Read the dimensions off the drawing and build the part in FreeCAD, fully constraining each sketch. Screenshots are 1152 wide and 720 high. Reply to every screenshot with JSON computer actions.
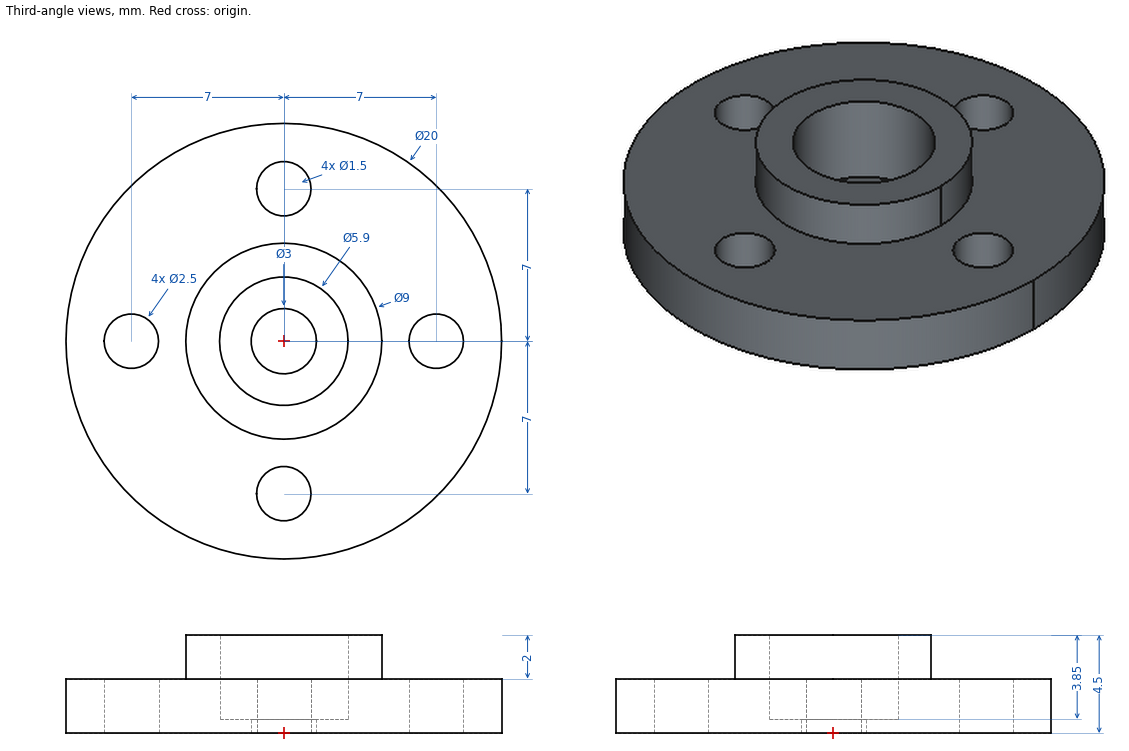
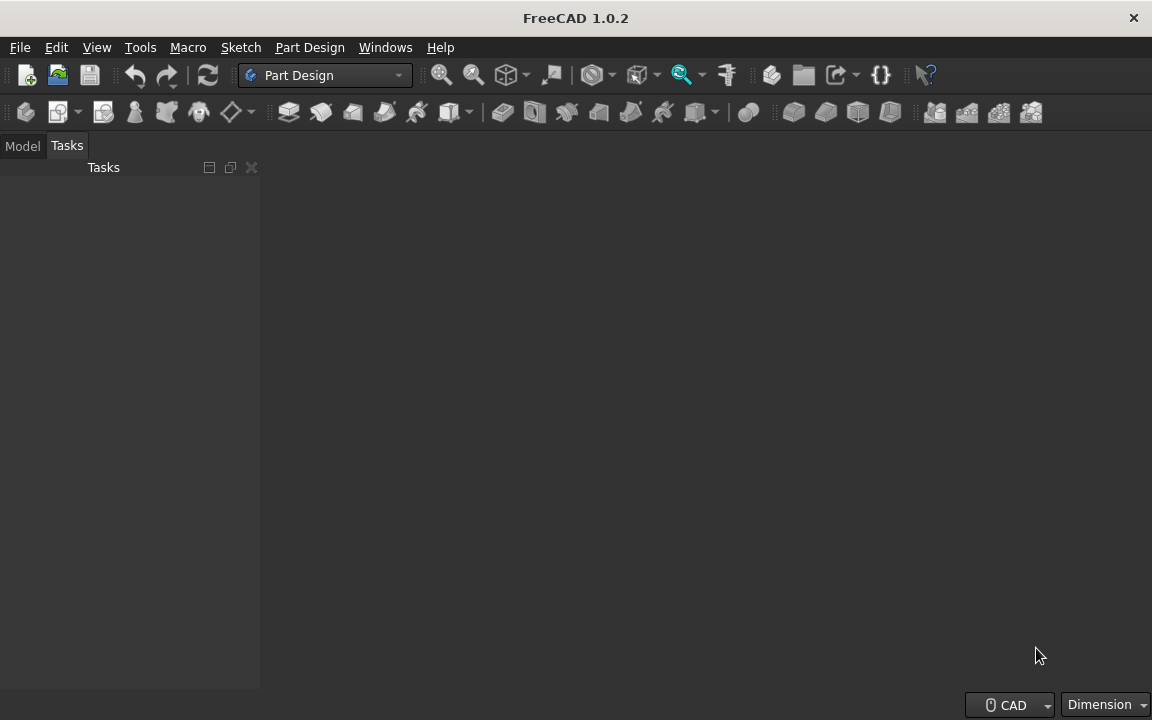
{"action": "left_click", "coordinate": [26, 76]}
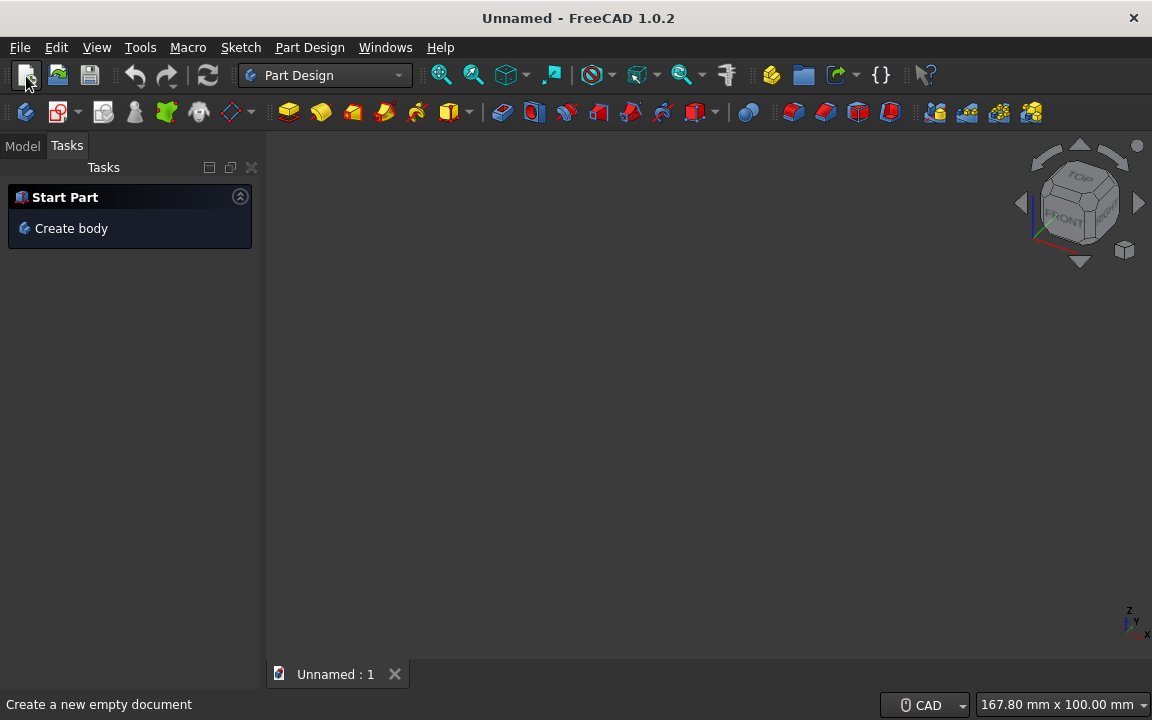
{"action": "left_click", "coordinate": [58, 112]}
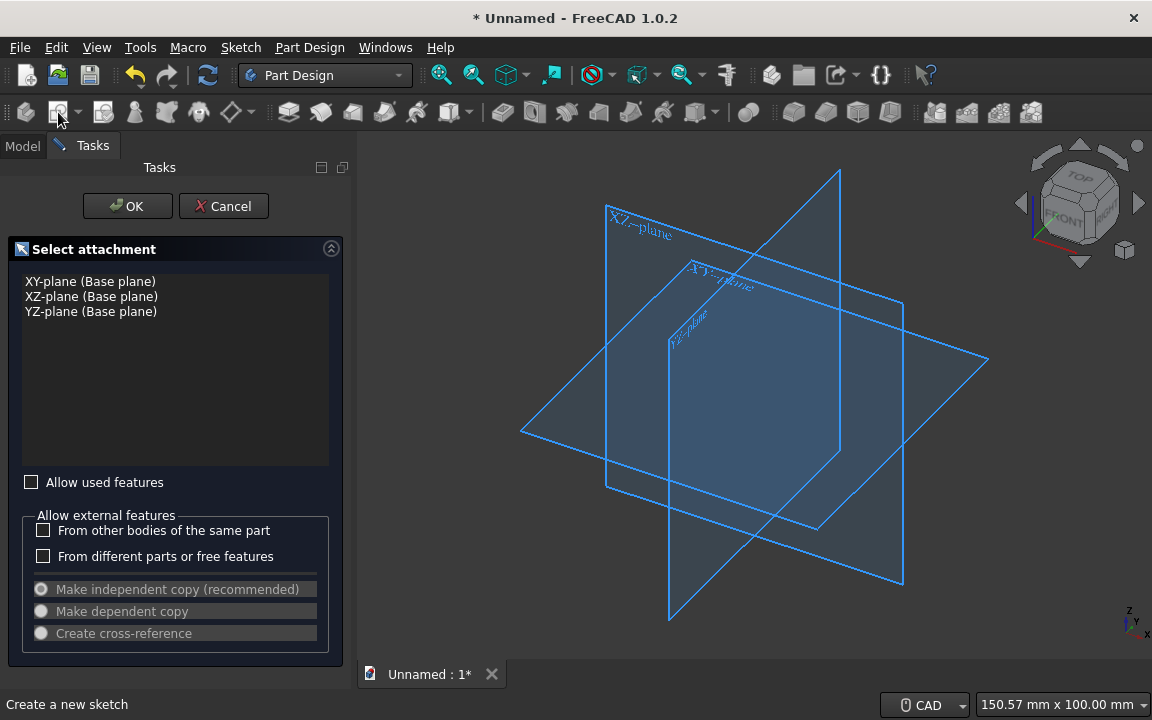
{"action": "left_click", "coordinate": [82, 282]}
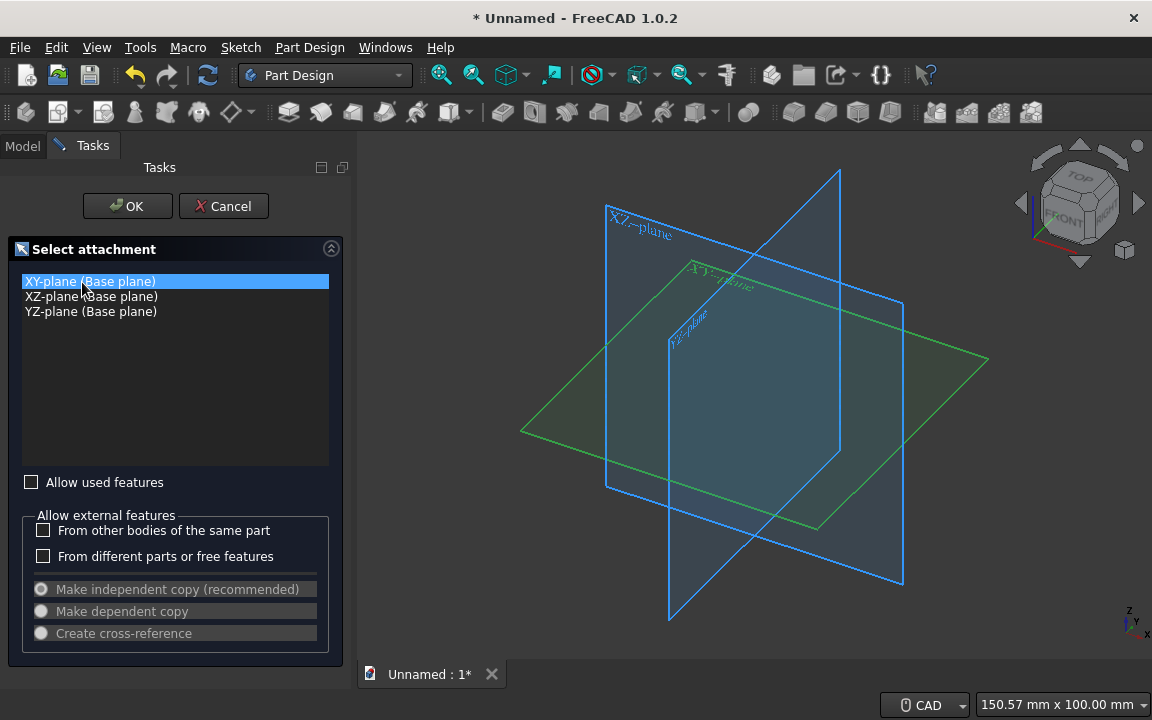
{"action": "left_click", "coordinate": [128, 206]}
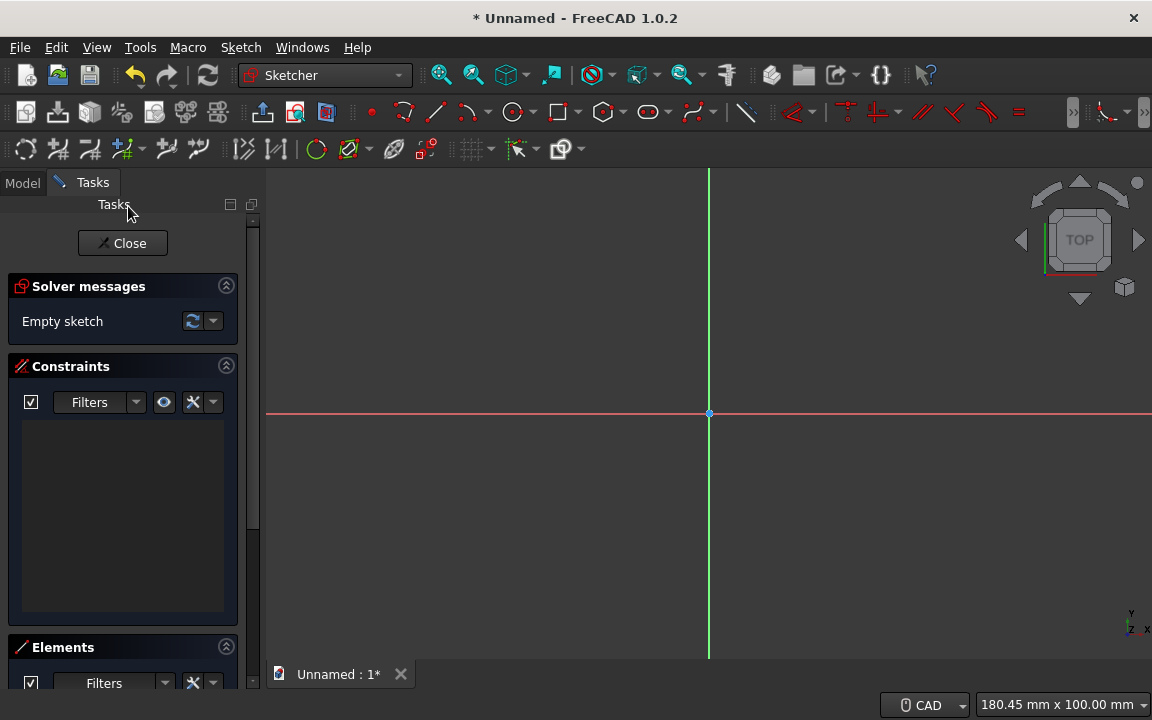
{"action": "scroll", "coordinate": [739, 414], "scroll_direction": "up", "scroll_amount": 6}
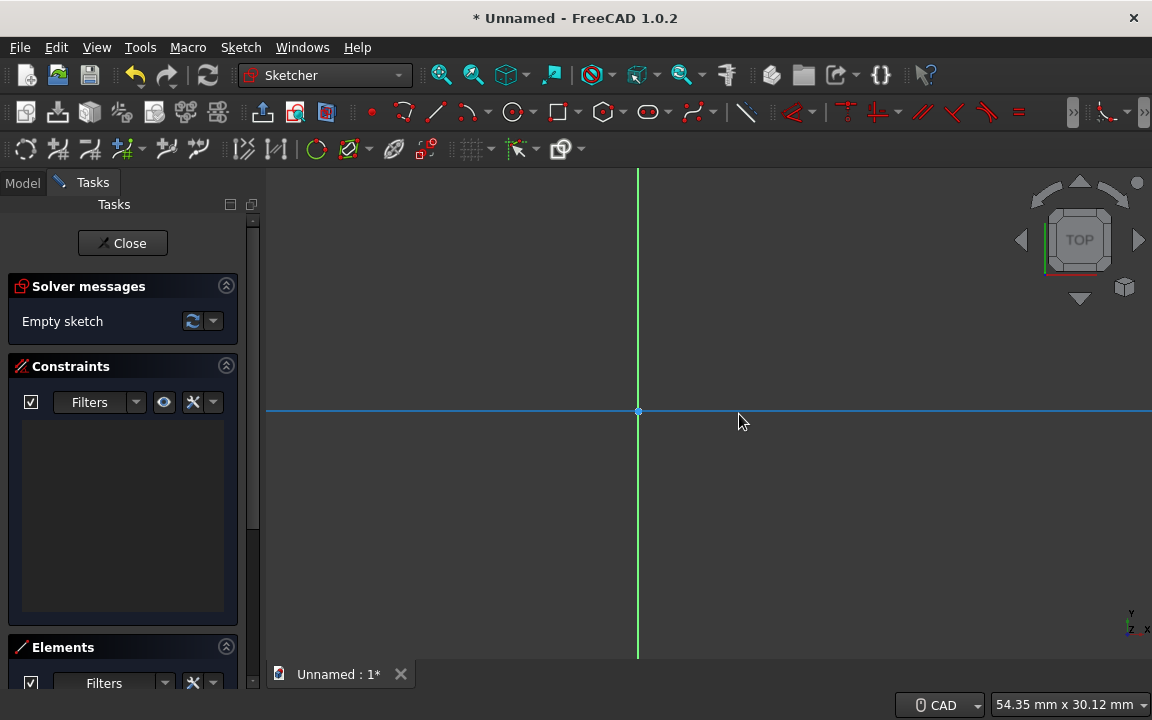
{"action": "key", "text": "g c"}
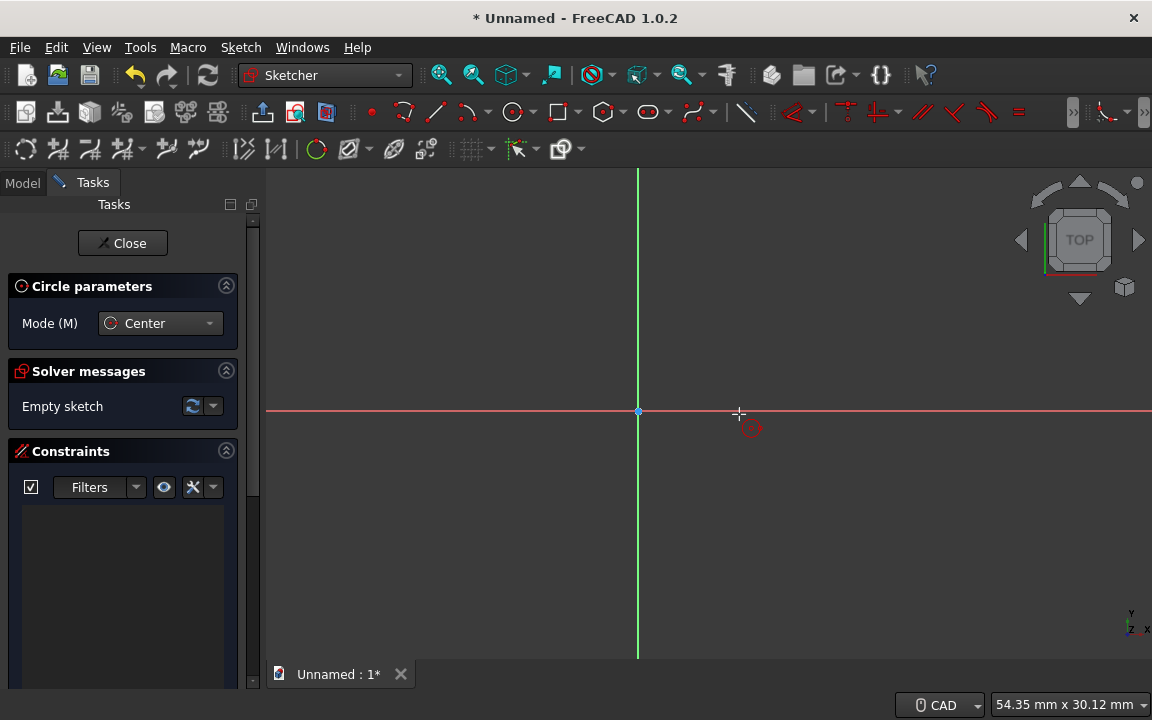
{"action": "left_click", "coordinate": [638, 411]}
{"action": "left_click", "coordinate": [753, 296]}
{"action": "key", "text": "Escape"}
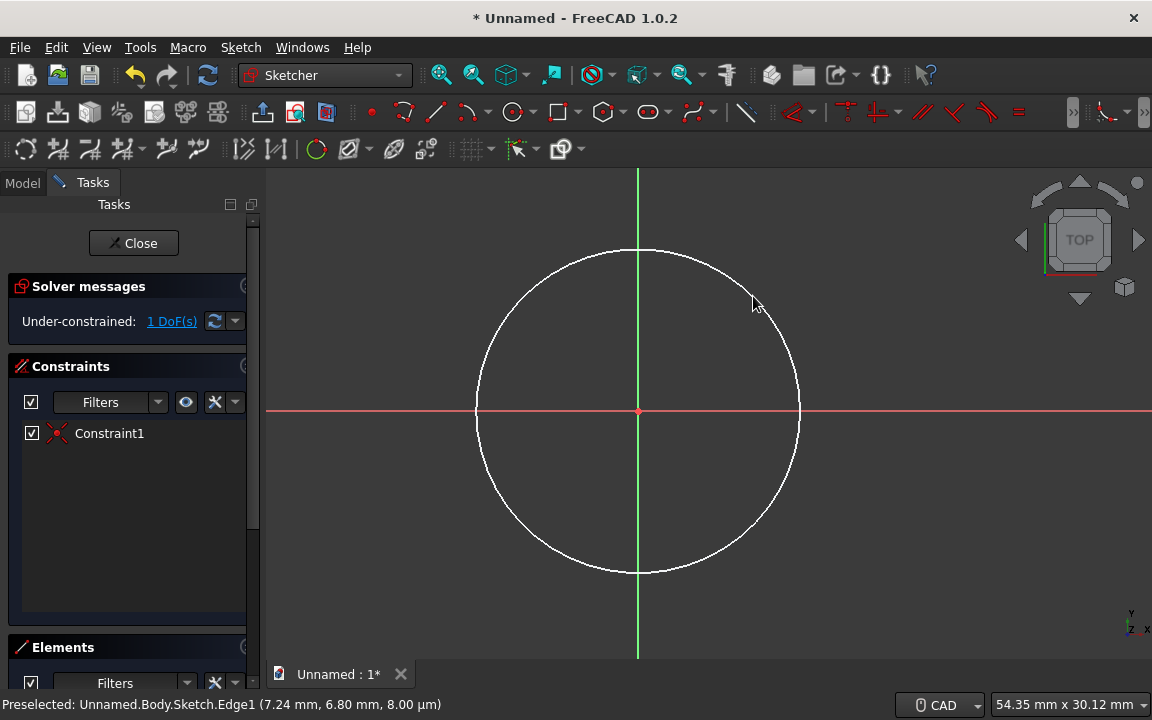
{"action": "key", "text": "d"}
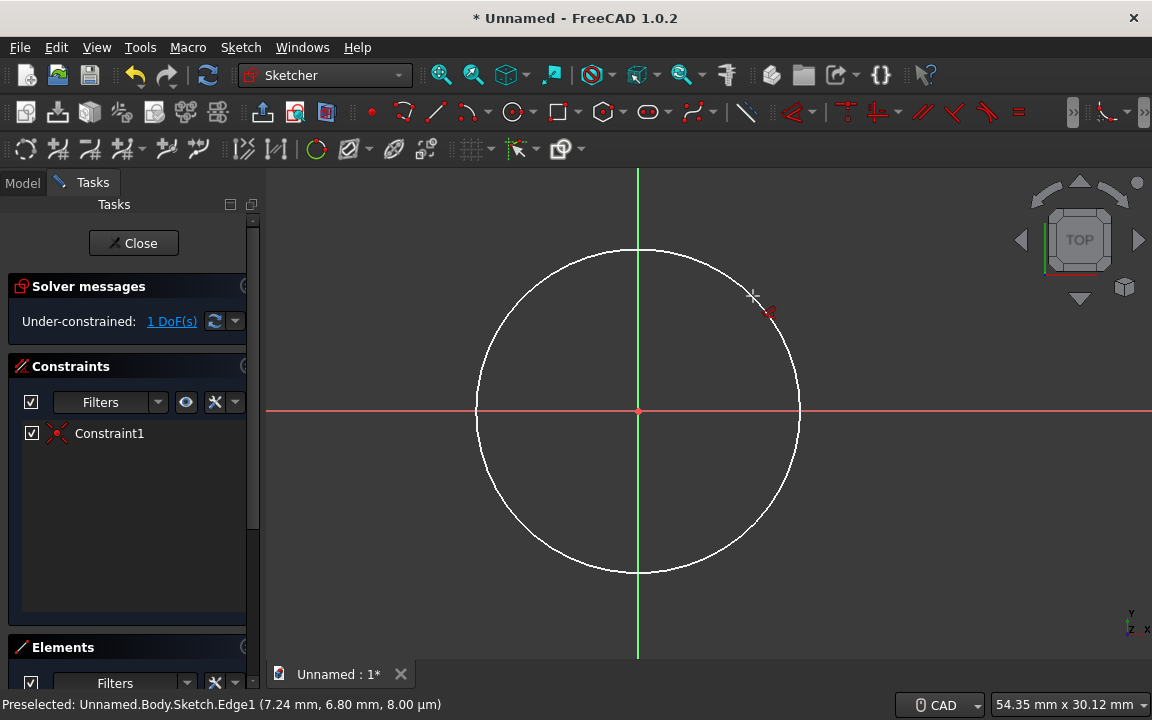
{"action": "left_click", "coordinate": [752, 296]}
{"action": "left_click", "coordinate": [774, 273]}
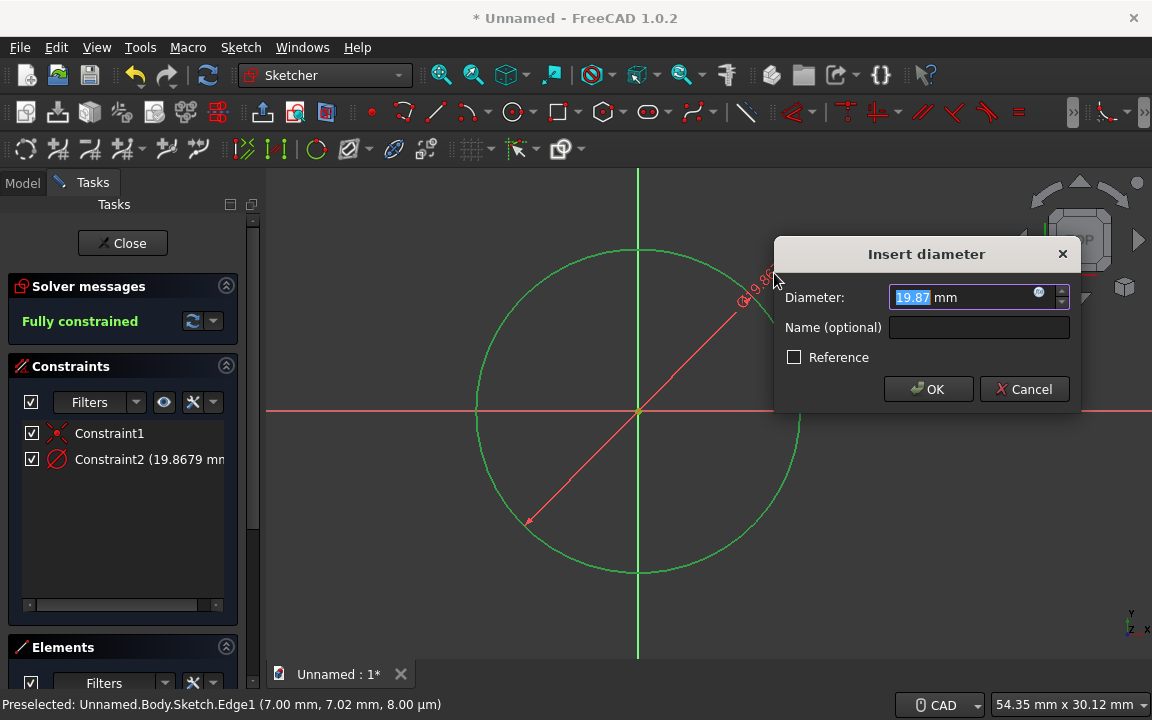
{"action": "type", "text": "20"}
{"action": "key", "text": "Return"}
{"action": "key", "text": "Escape"}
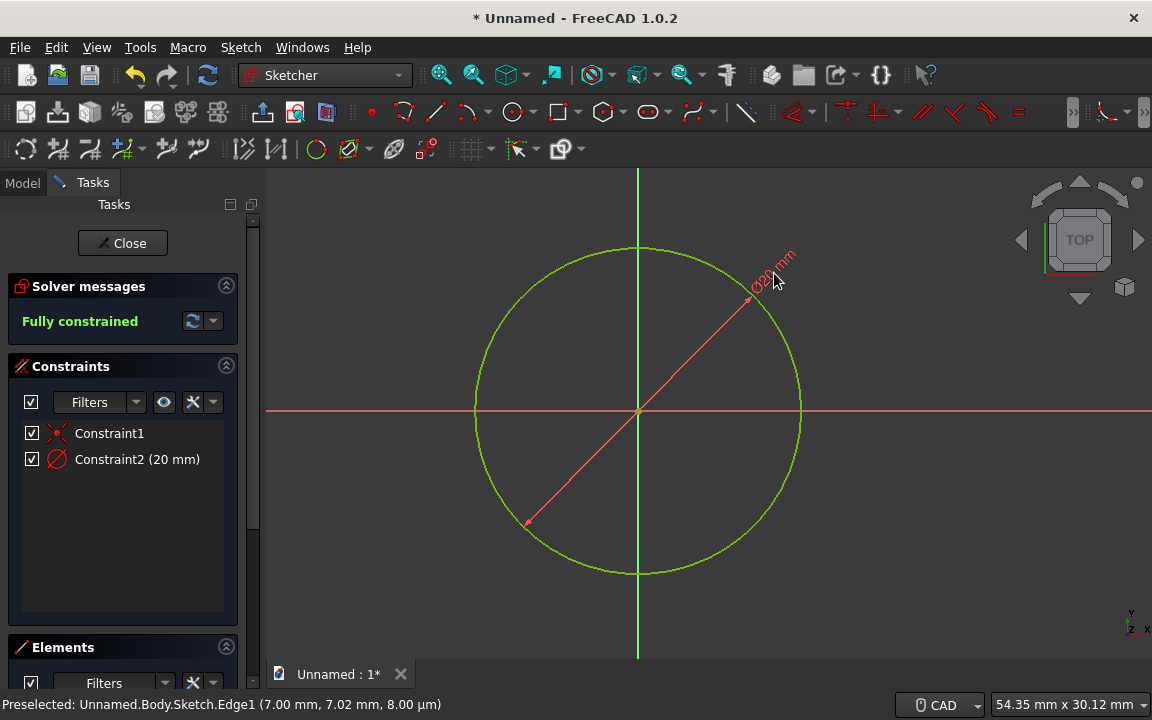
{"action": "left_click", "coordinate": [123, 243]}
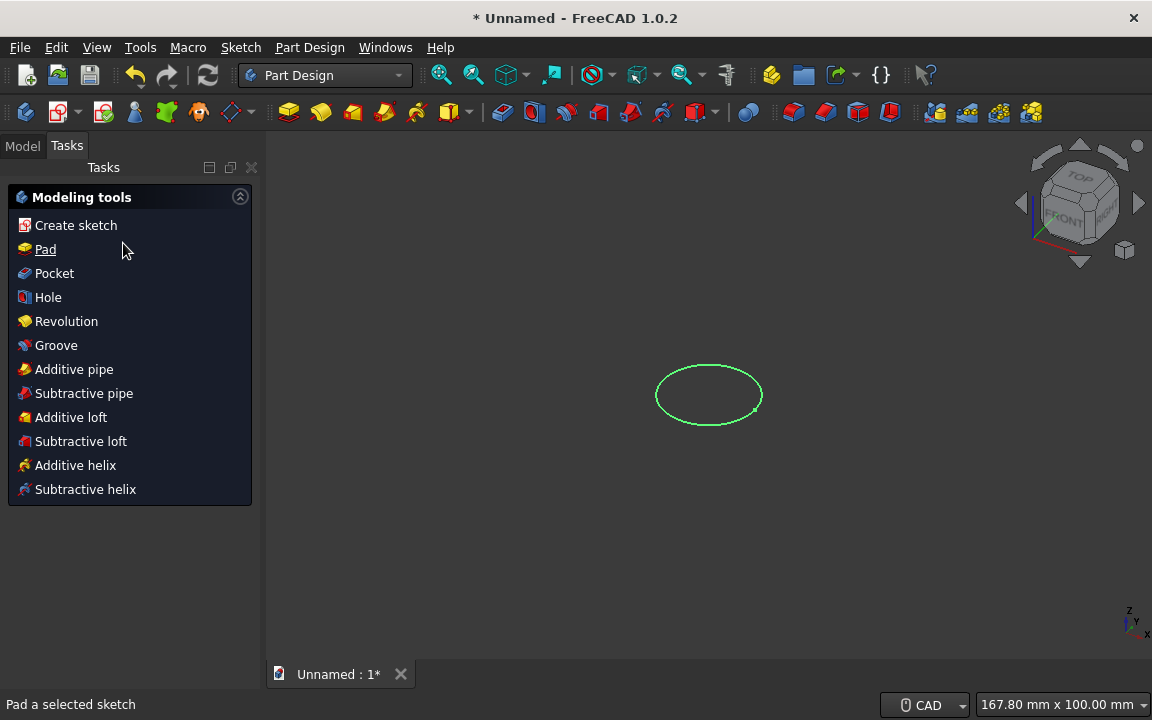
{"action": "left_click", "coordinate": [290, 112]}